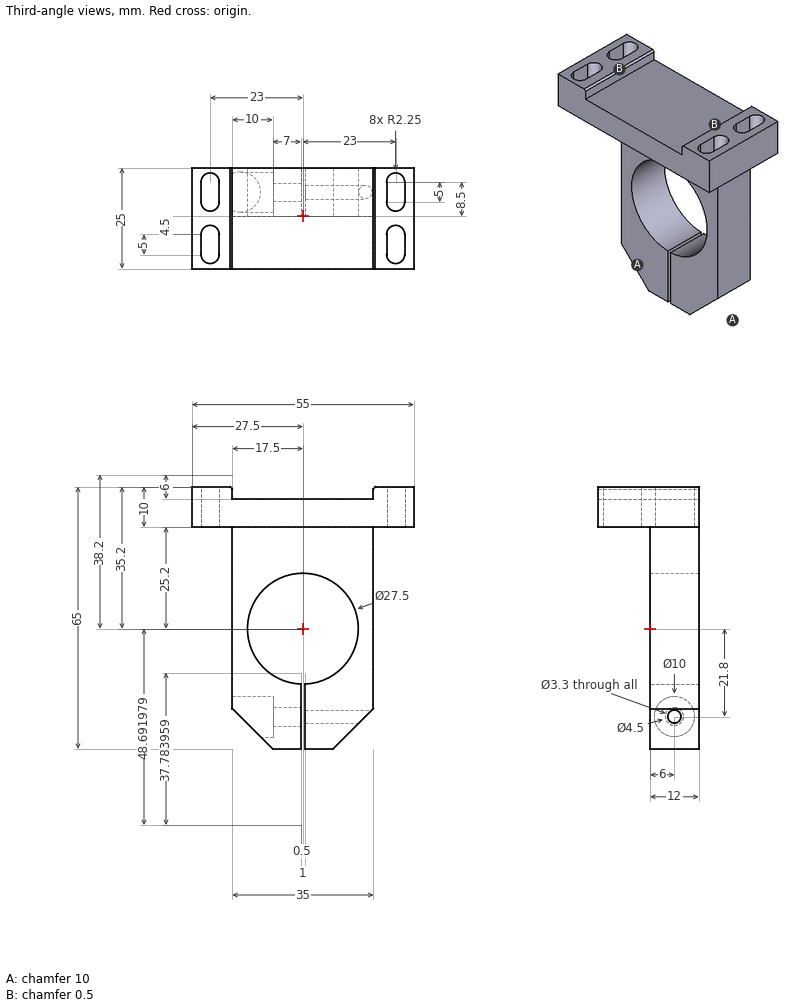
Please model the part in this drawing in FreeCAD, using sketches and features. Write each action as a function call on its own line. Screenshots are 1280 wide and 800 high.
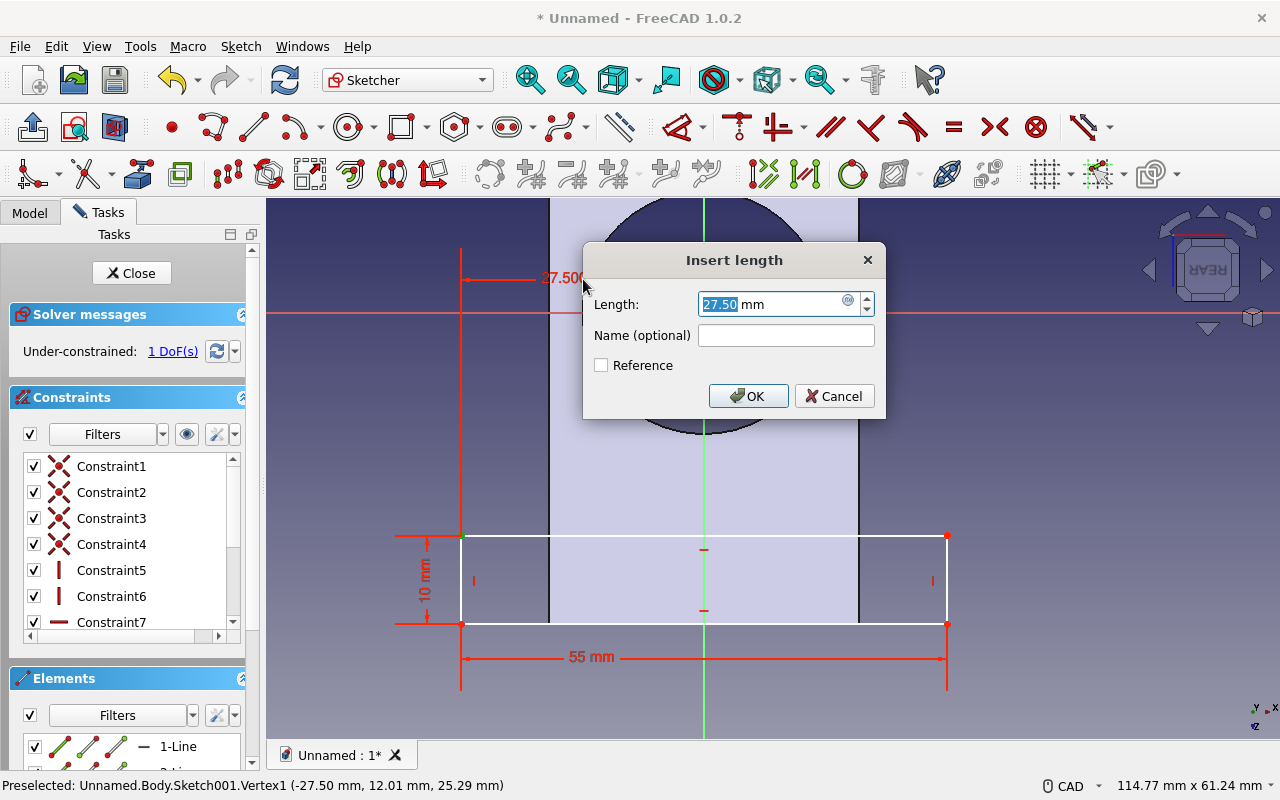
text(27.5)
key(Return)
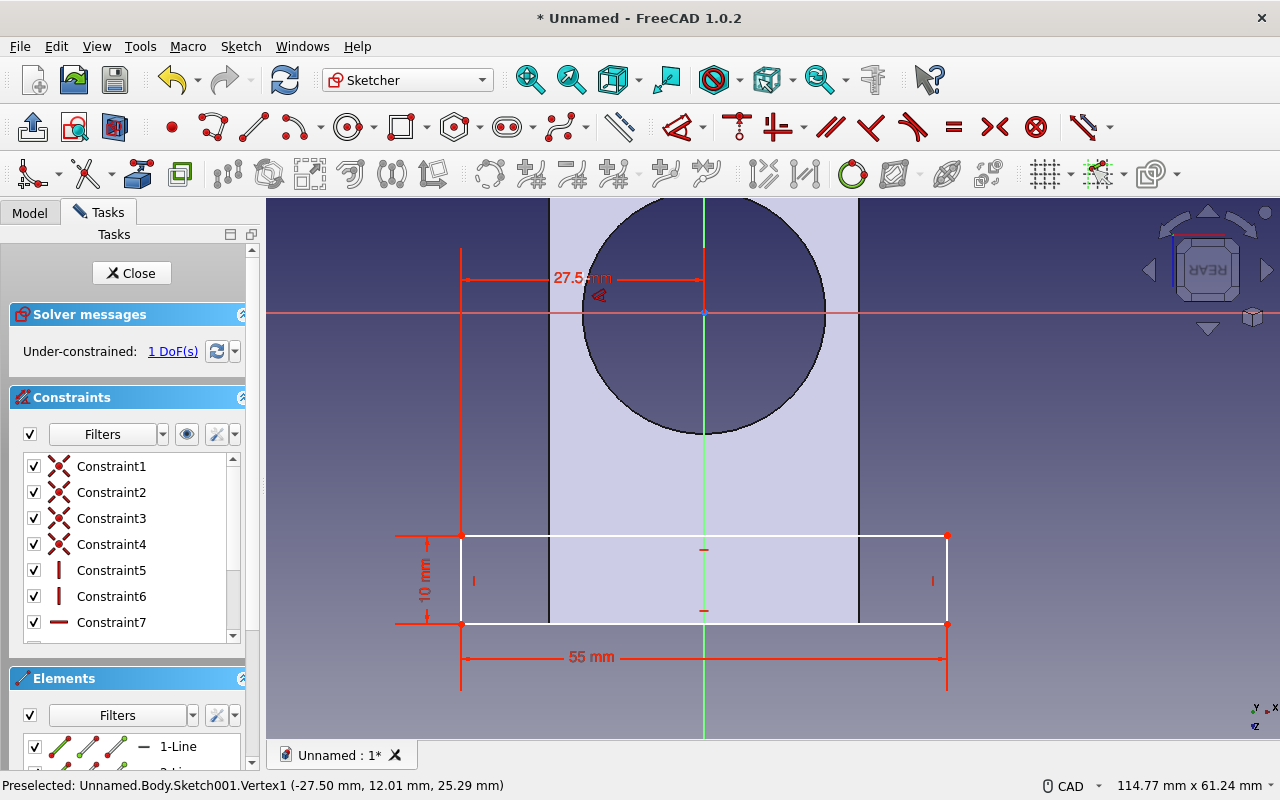
click(461, 536)
click(427, 424)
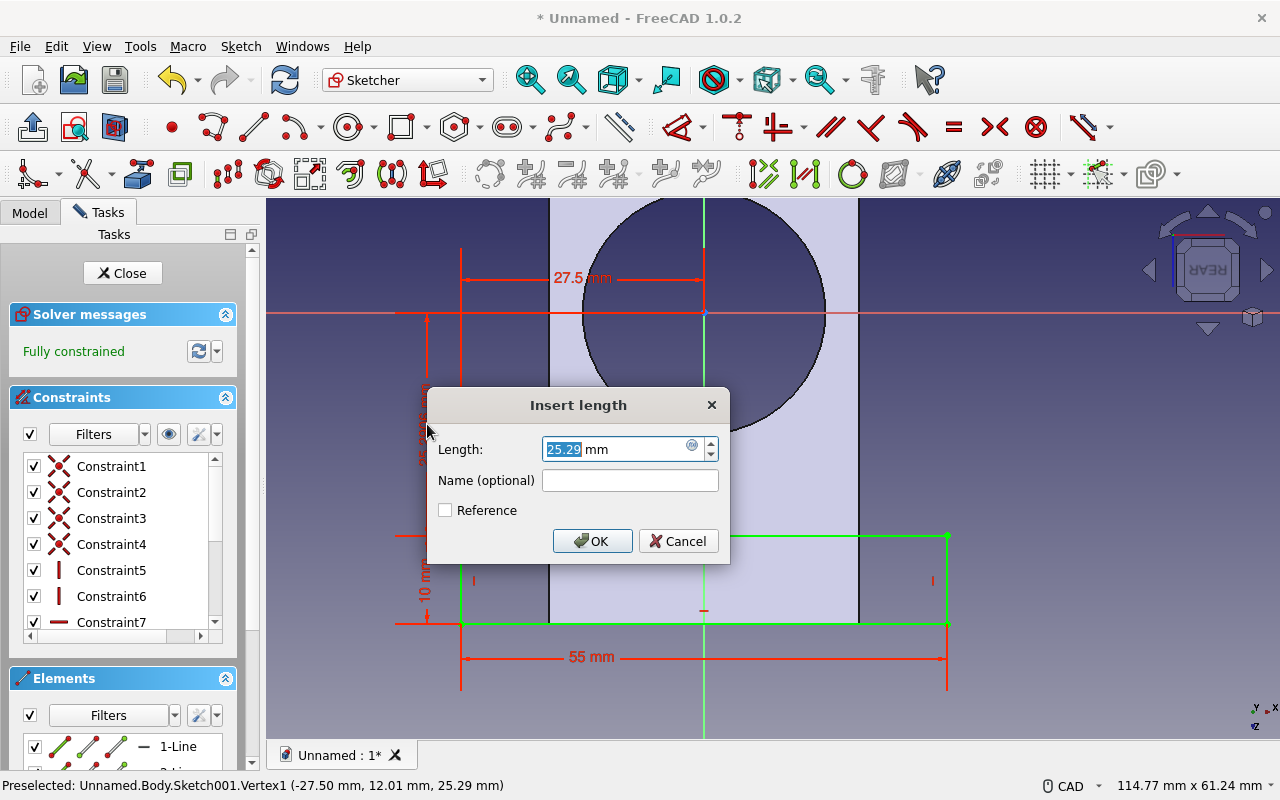
text(25.2)
key(Return)
key(Escape)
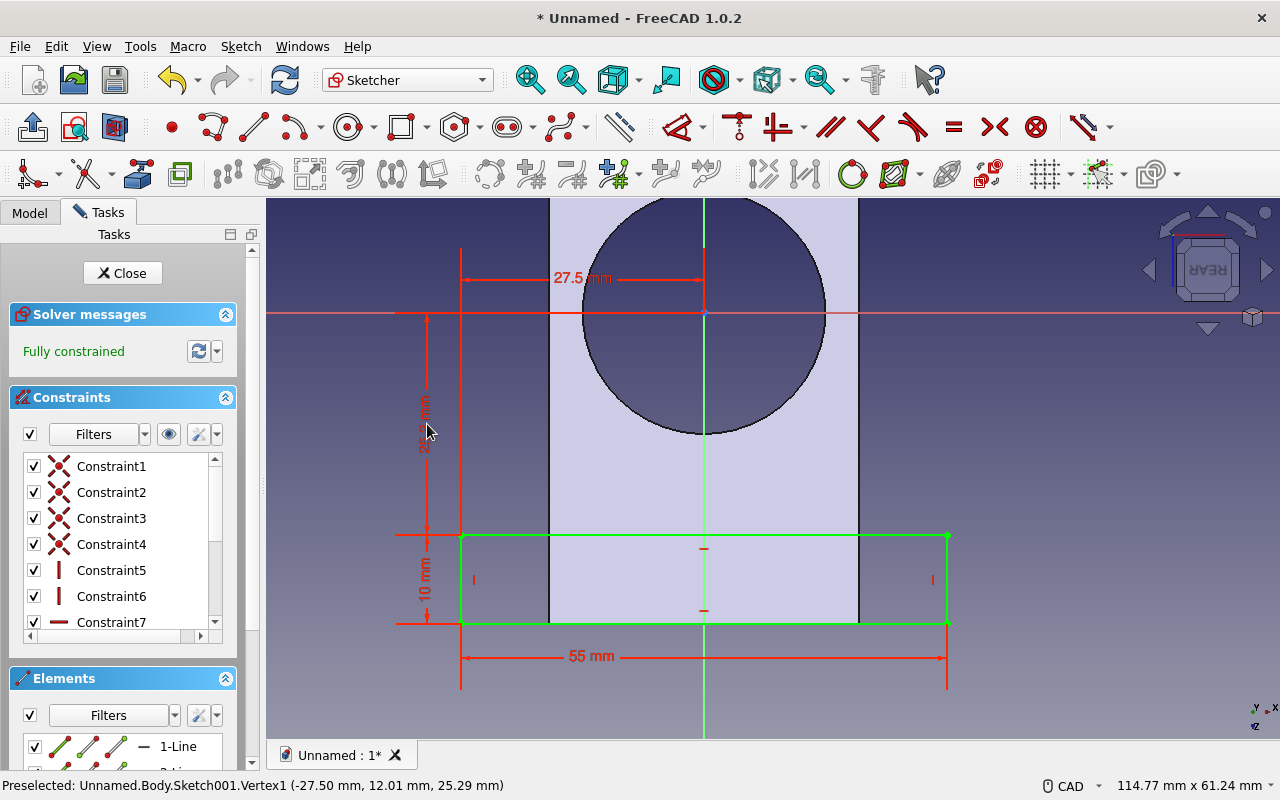
click(123, 273)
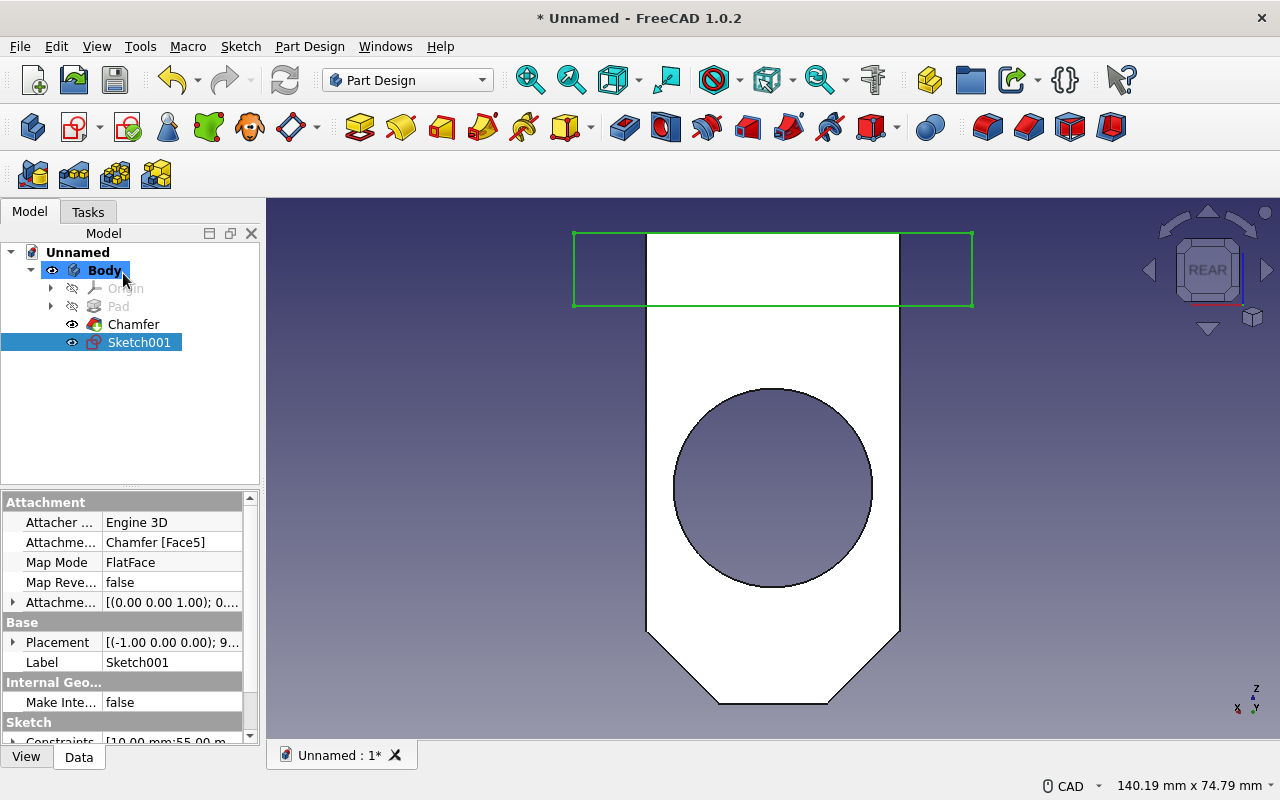
click(360, 128)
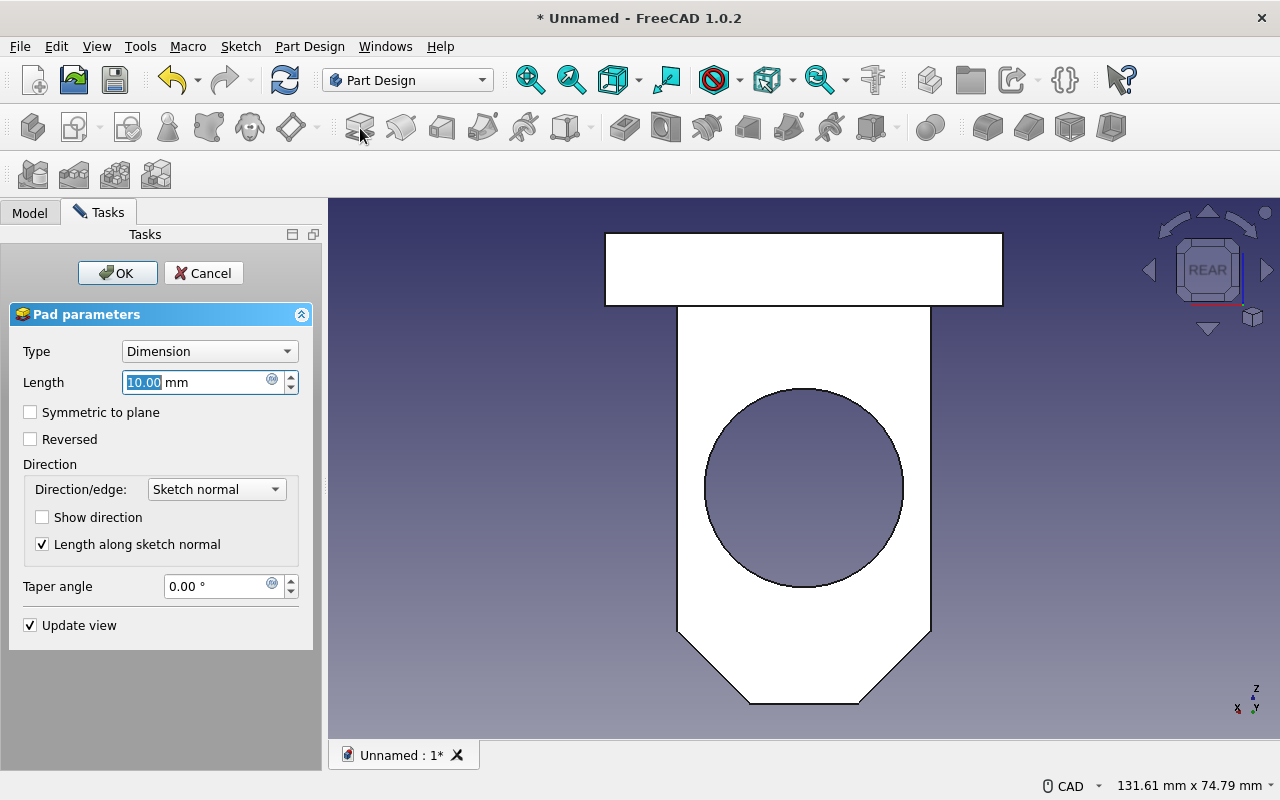
text(25)
key(Tab)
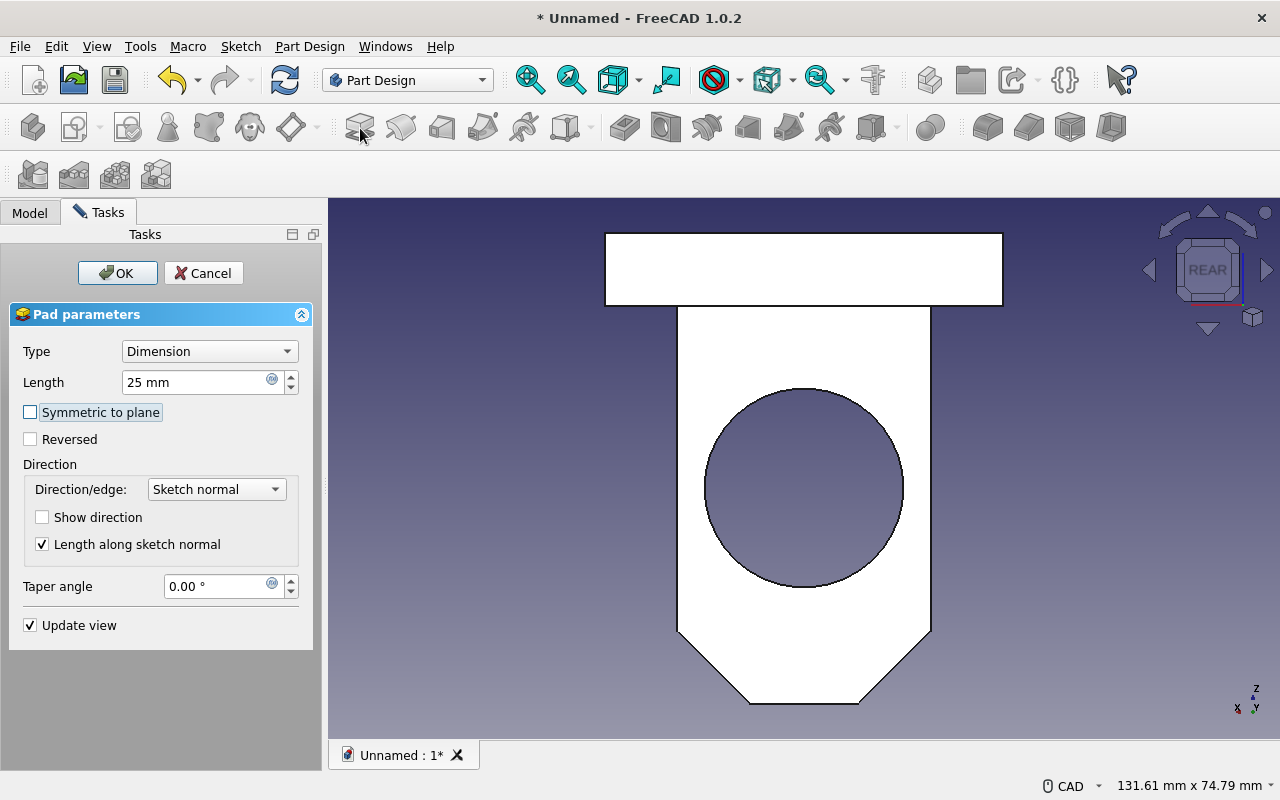
click(31, 439)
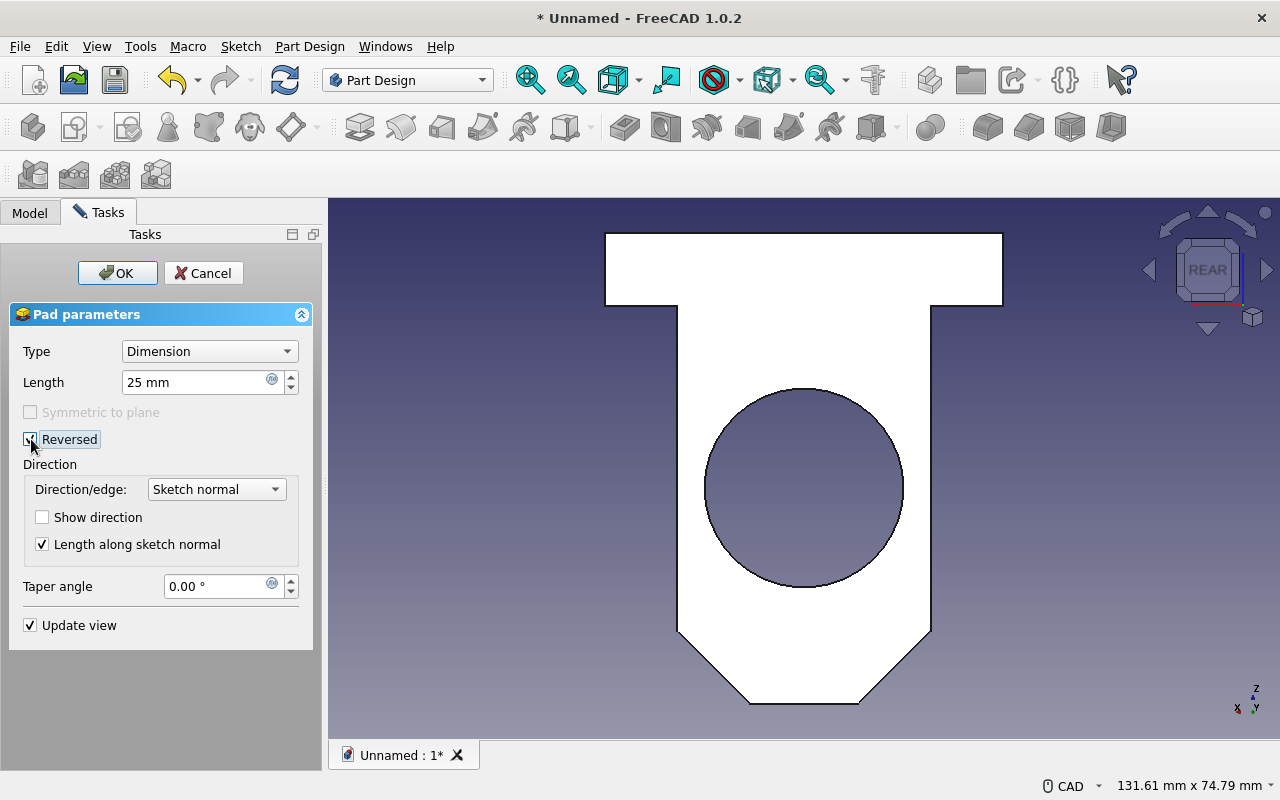
click(118, 273)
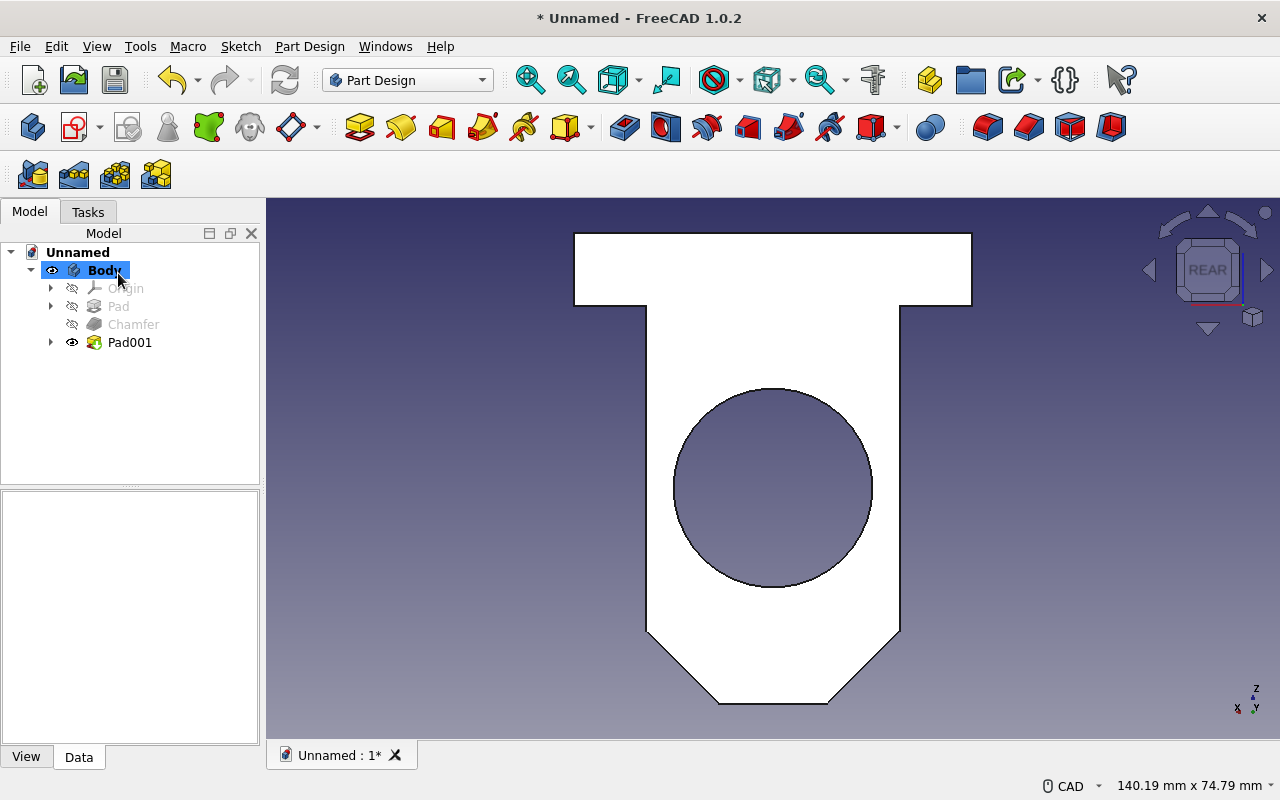
key(0)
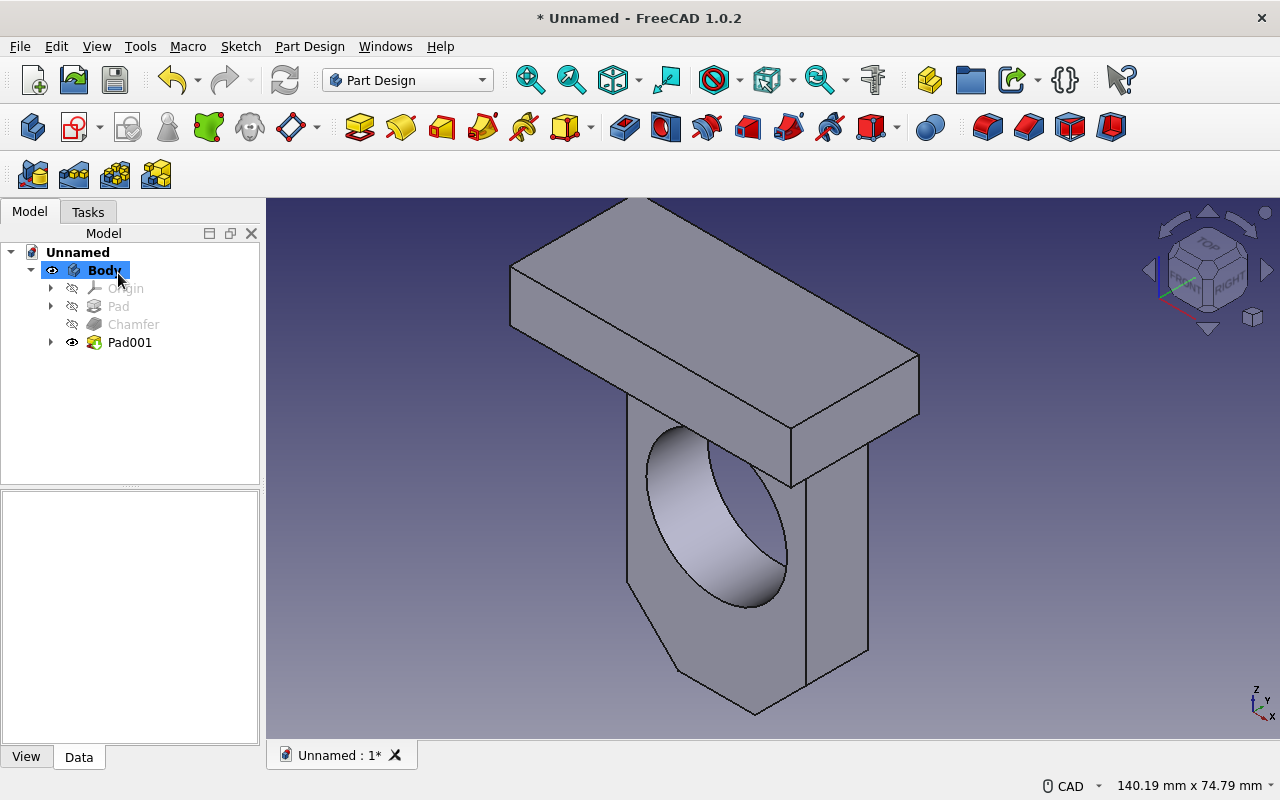
key(v)
key(f)